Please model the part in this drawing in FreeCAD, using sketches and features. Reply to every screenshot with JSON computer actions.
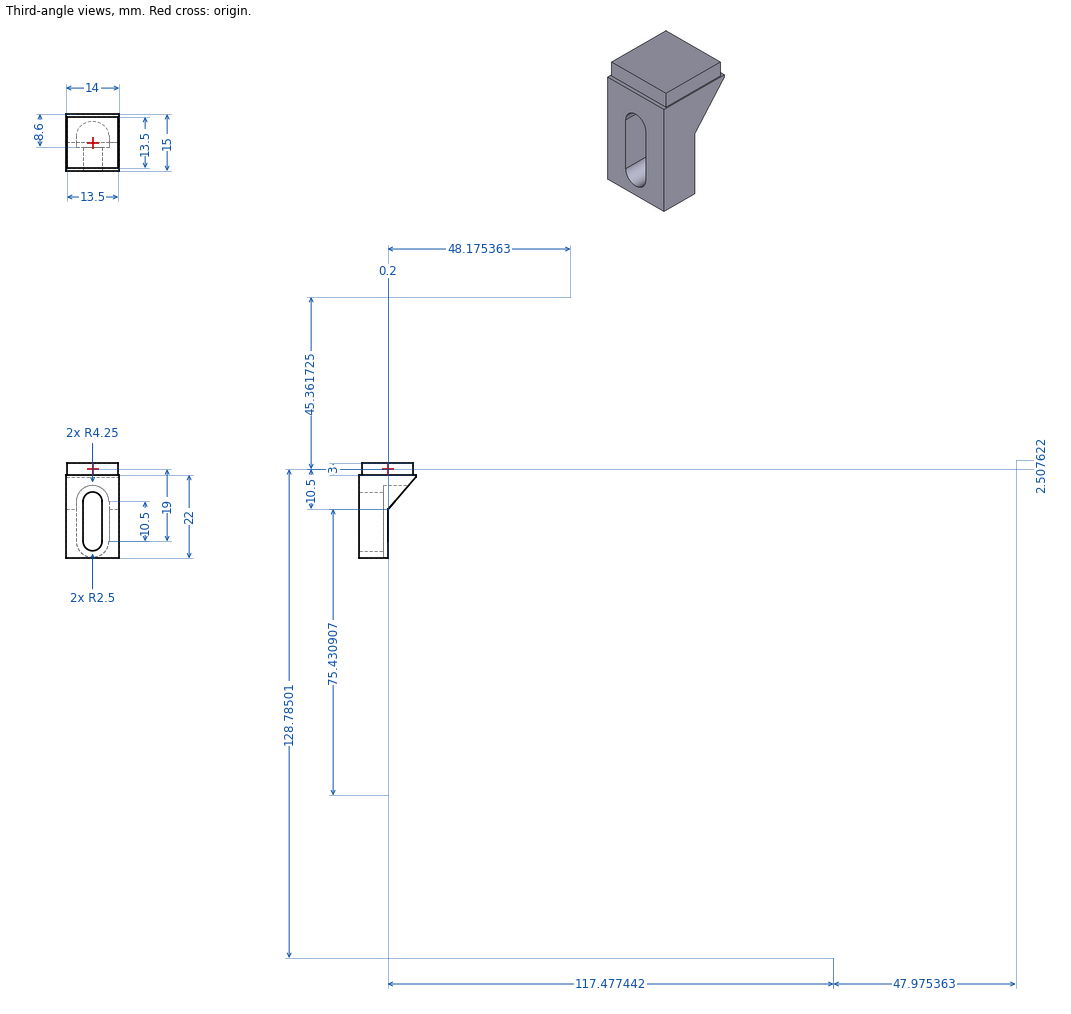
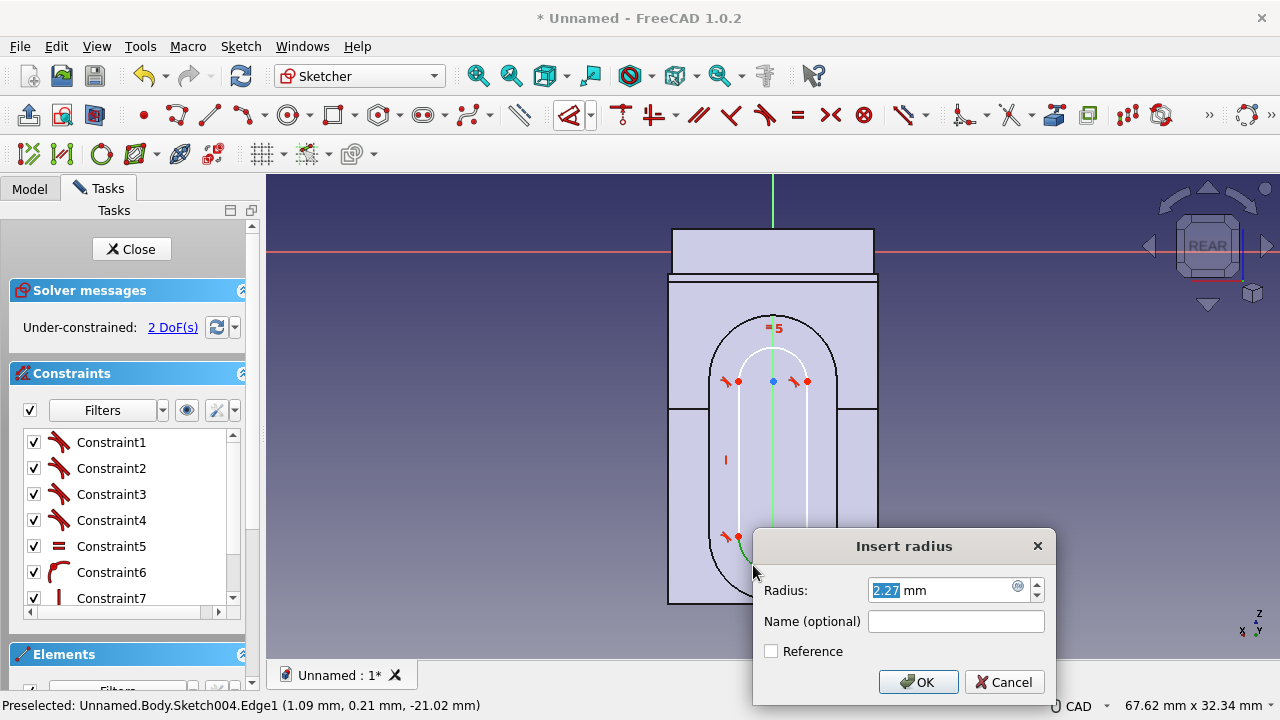
{"action": "type", "text": "2.5"}
{"action": "key", "text": "Return"}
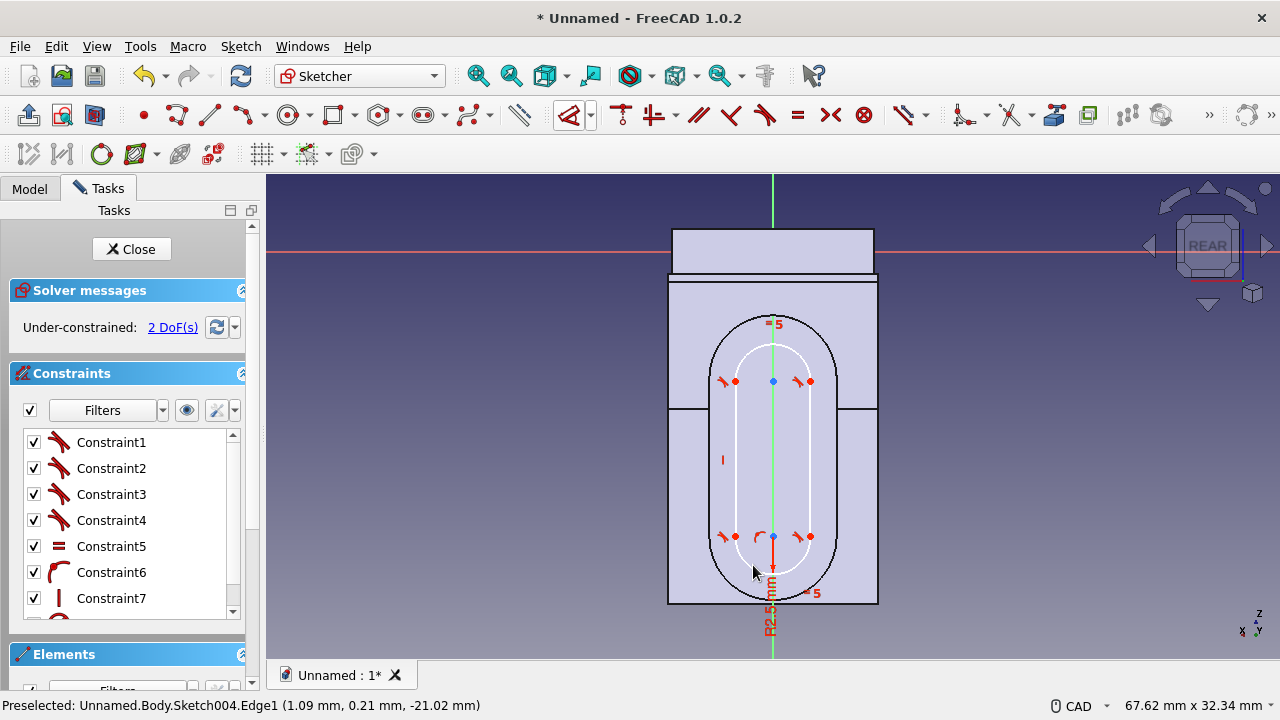
{"action": "left_click", "coordinate": [736, 537]}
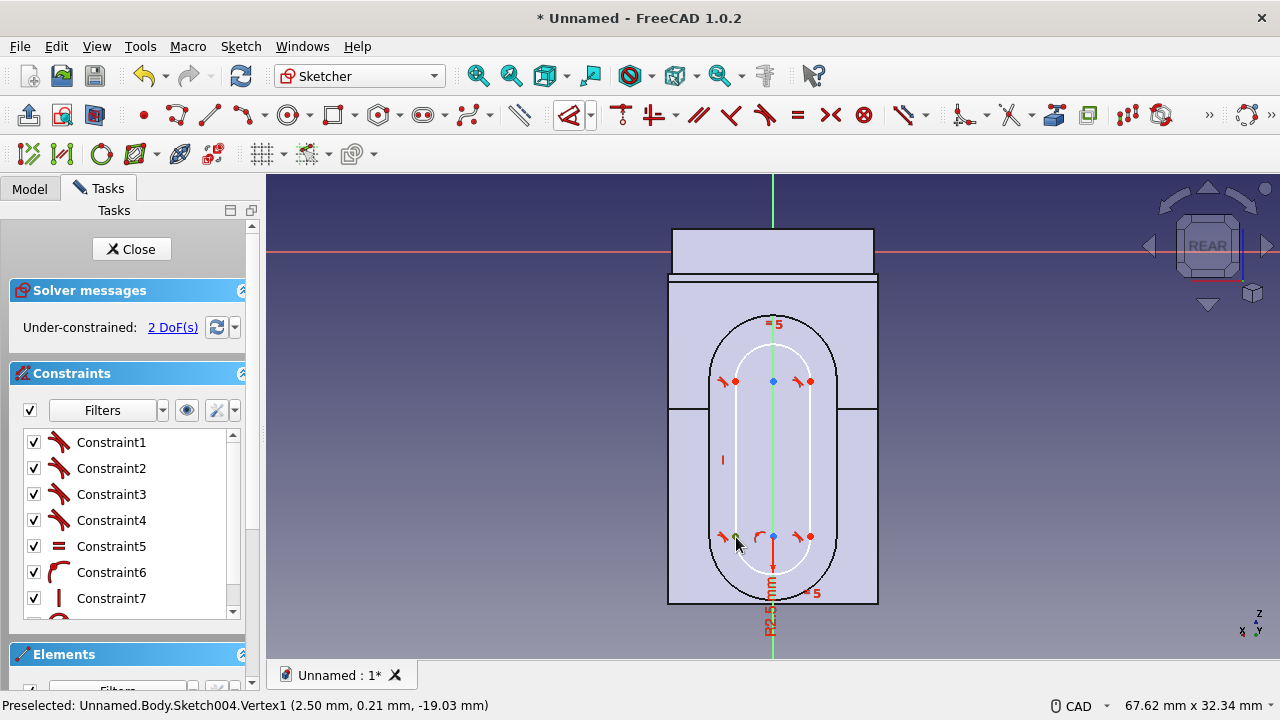
{"action": "key", "text": "i"}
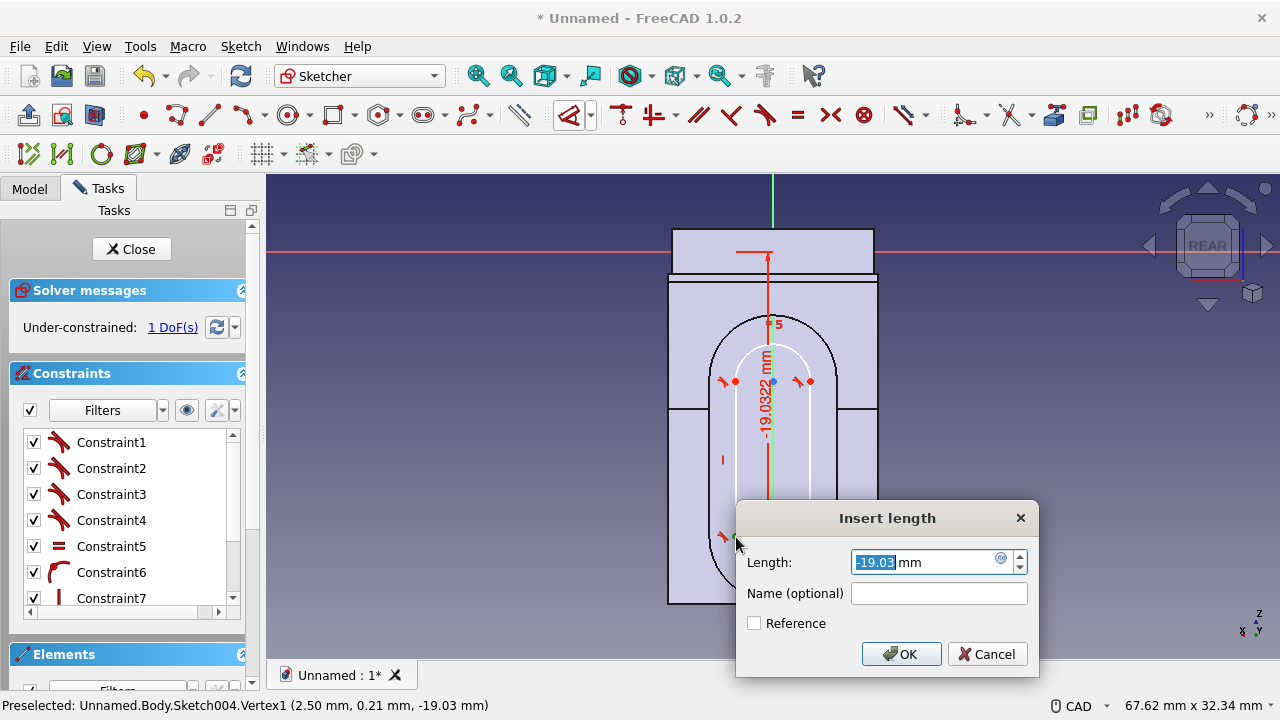
{"action": "type", "text": "-19"}
{"action": "key", "text": "Return"}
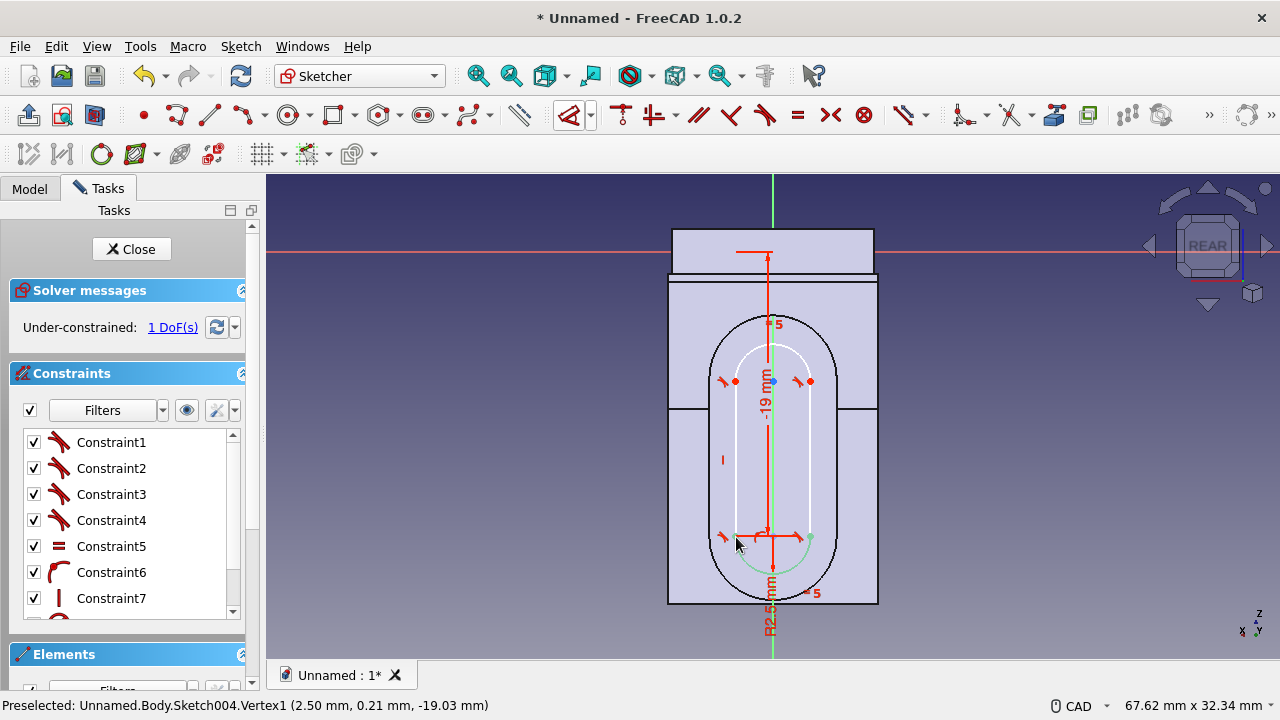
{"action": "left_click", "coordinate": [736, 490]}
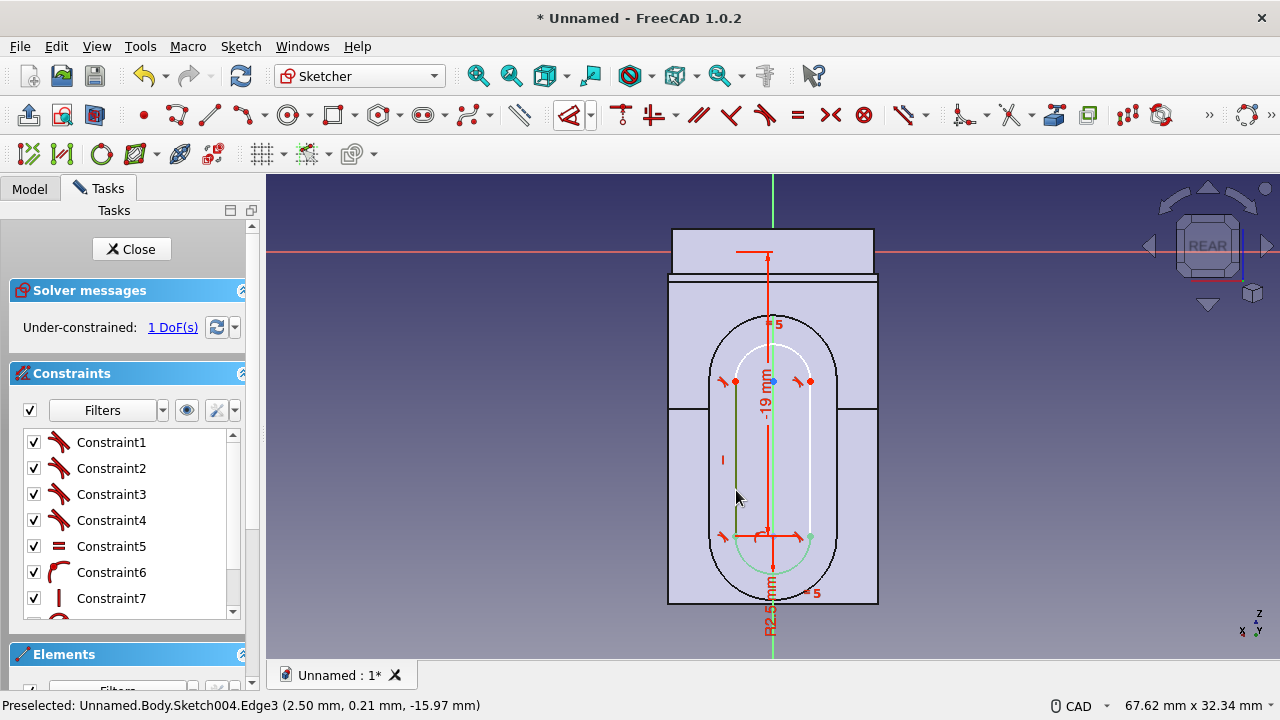
{"action": "key", "text": "i"}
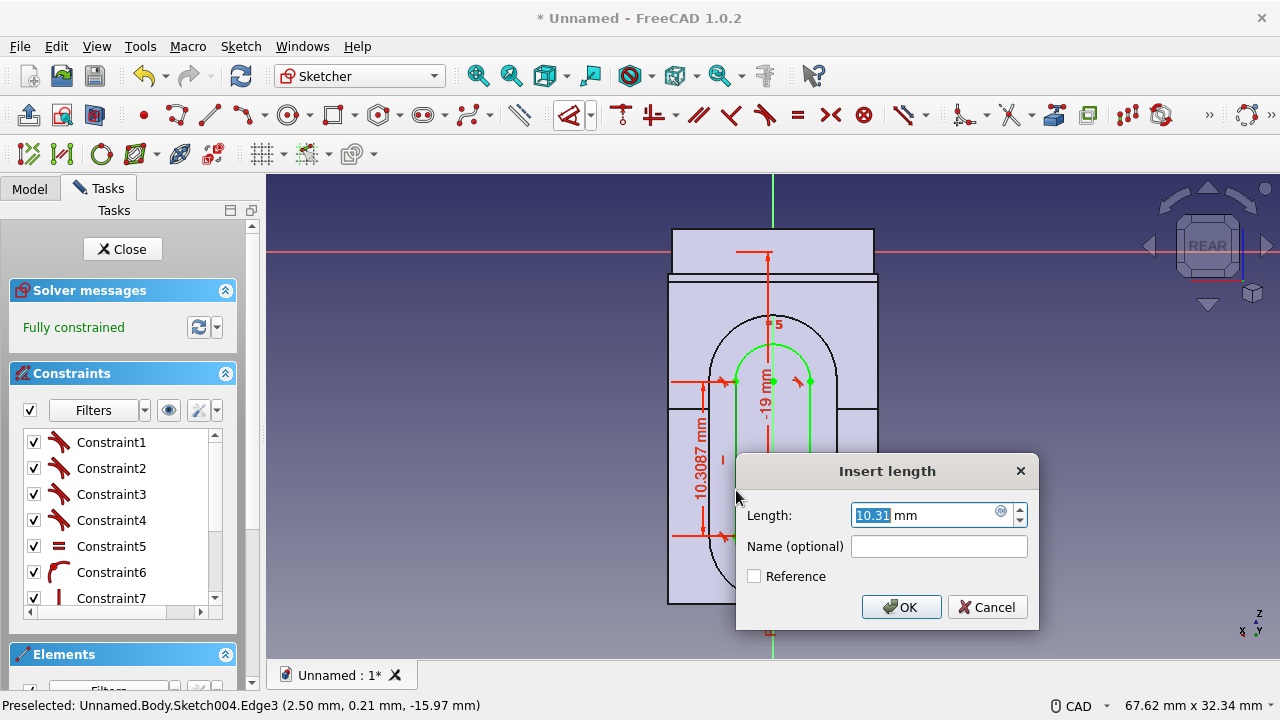
{"action": "type", "text": "10.5"}
{"action": "key", "text": "Return"}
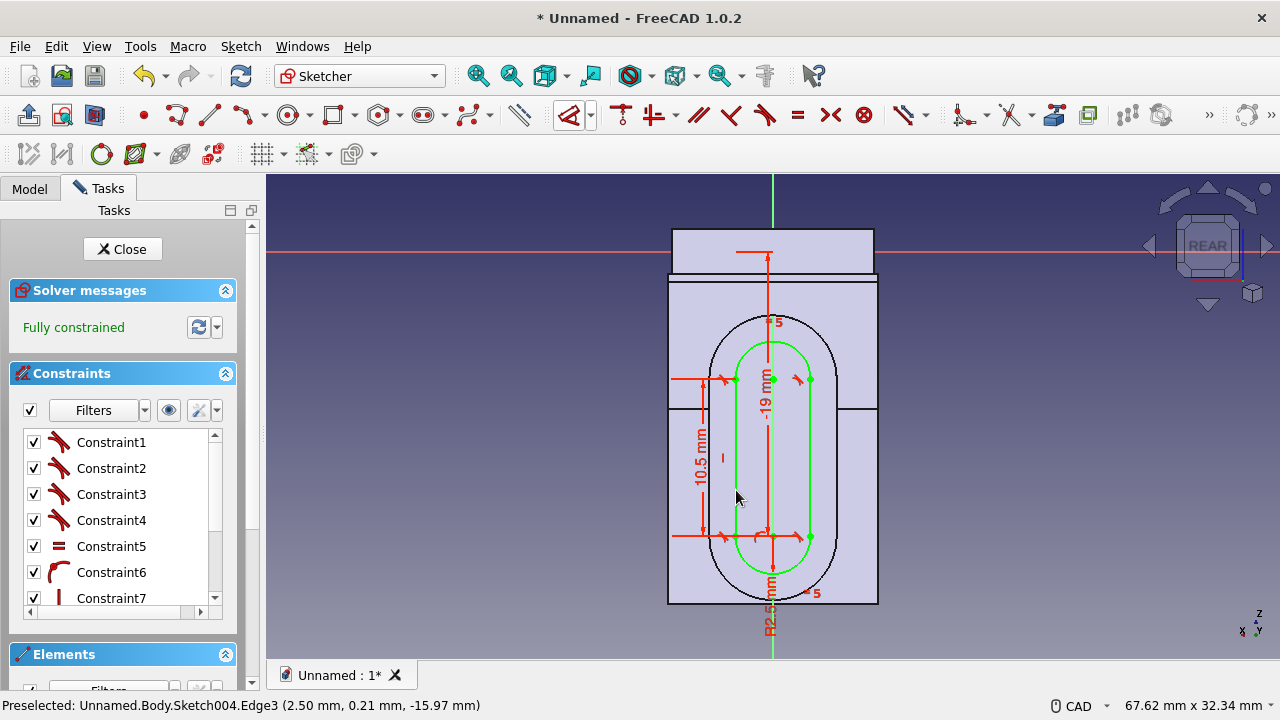
{"action": "left_click", "coordinate": [123, 249]}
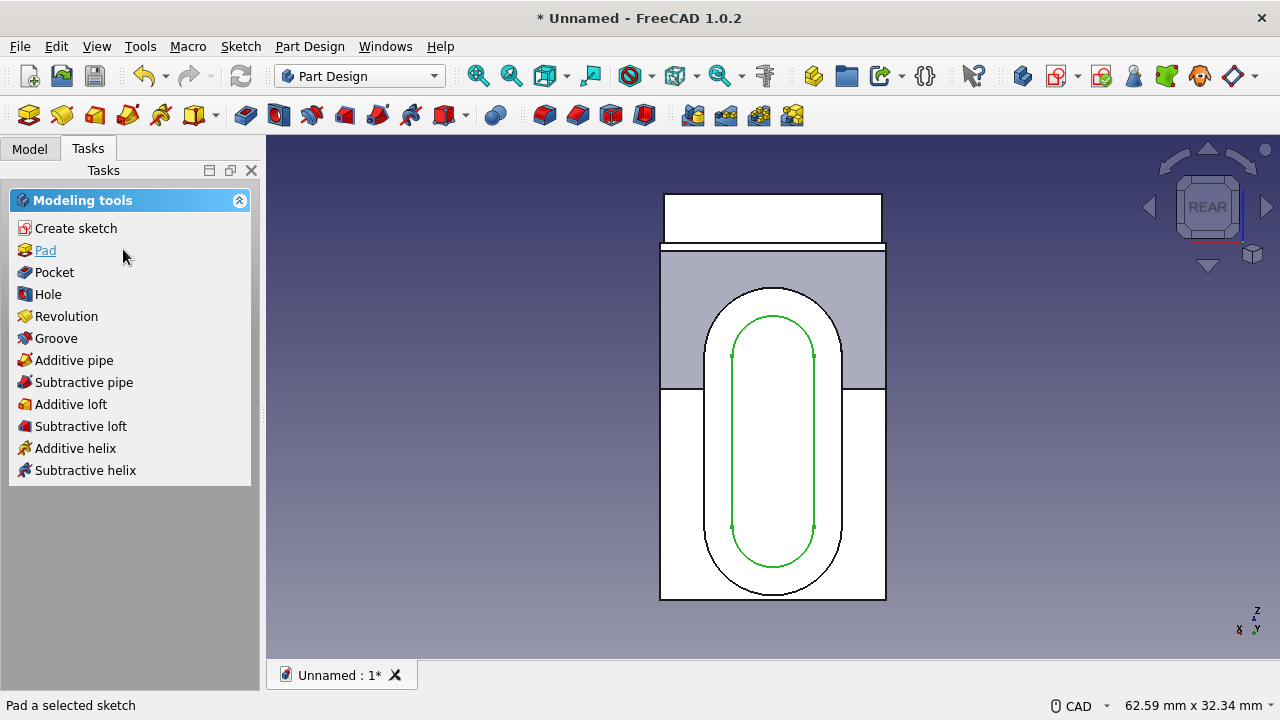
{"action": "left_click", "coordinate": [246, 116]}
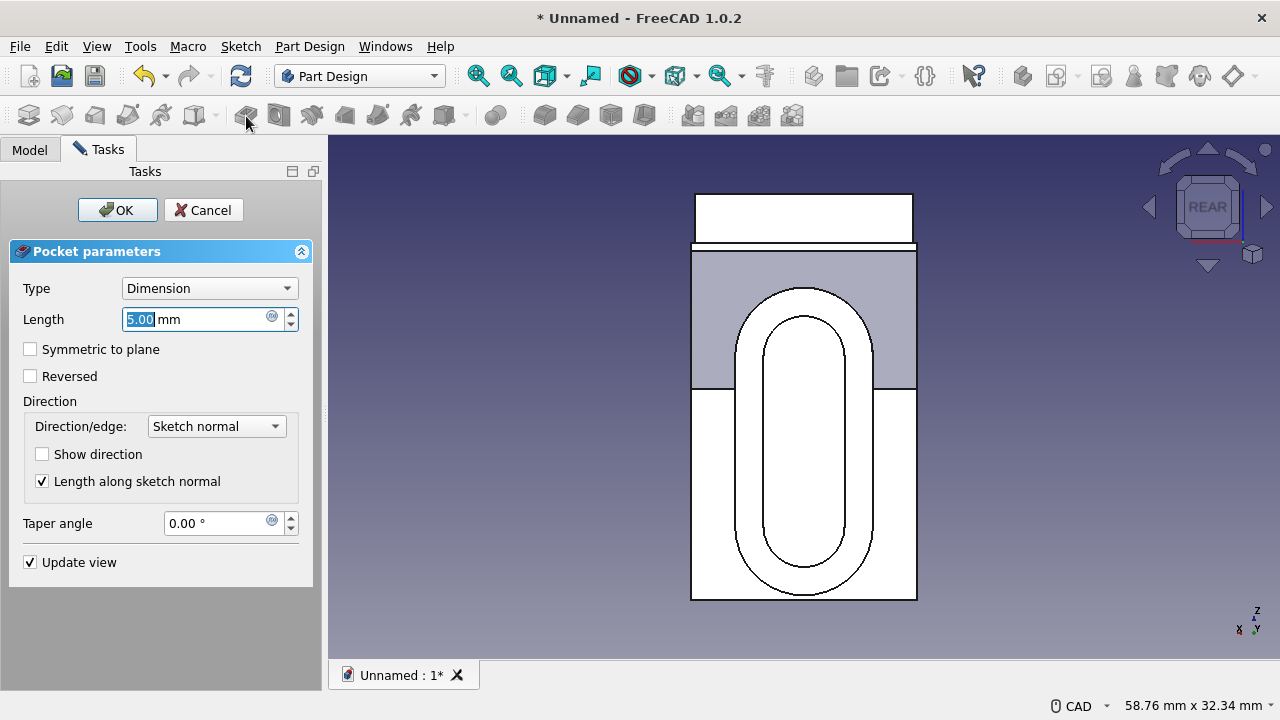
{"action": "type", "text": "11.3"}
{"action": "key", "text": "Tab"}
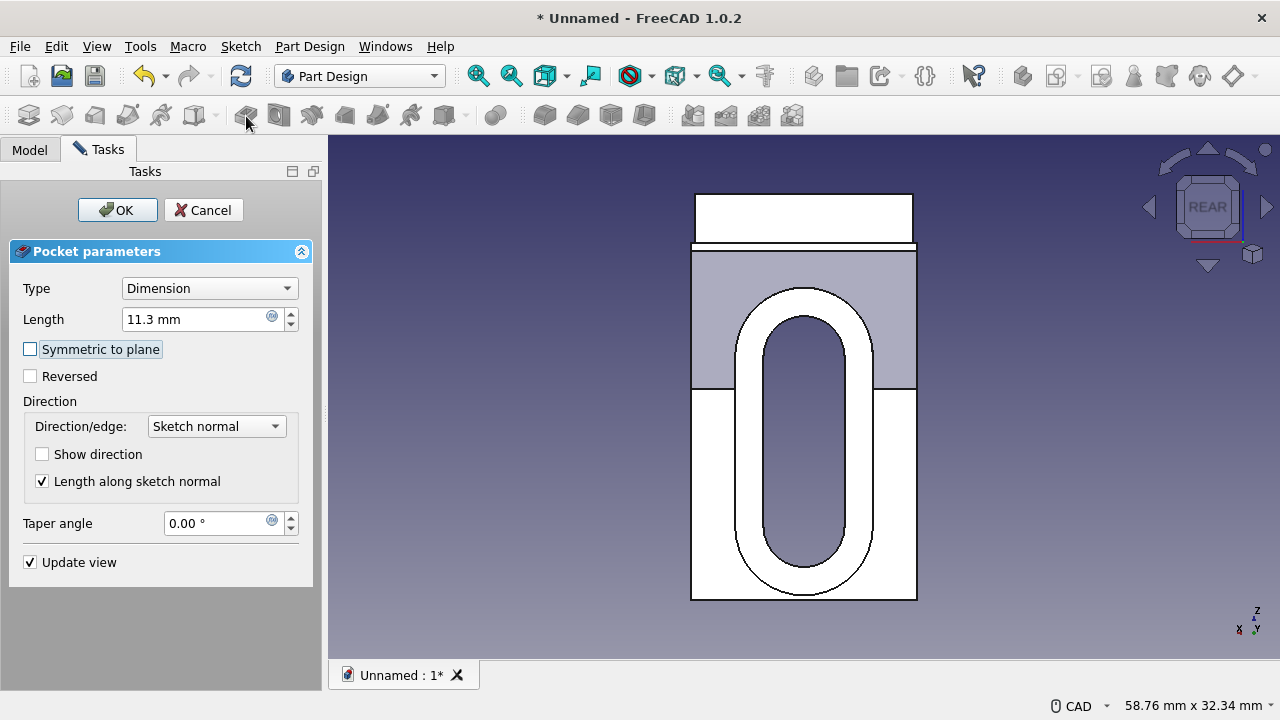
{"action": "left_click", "coordinate": [118, 210]}